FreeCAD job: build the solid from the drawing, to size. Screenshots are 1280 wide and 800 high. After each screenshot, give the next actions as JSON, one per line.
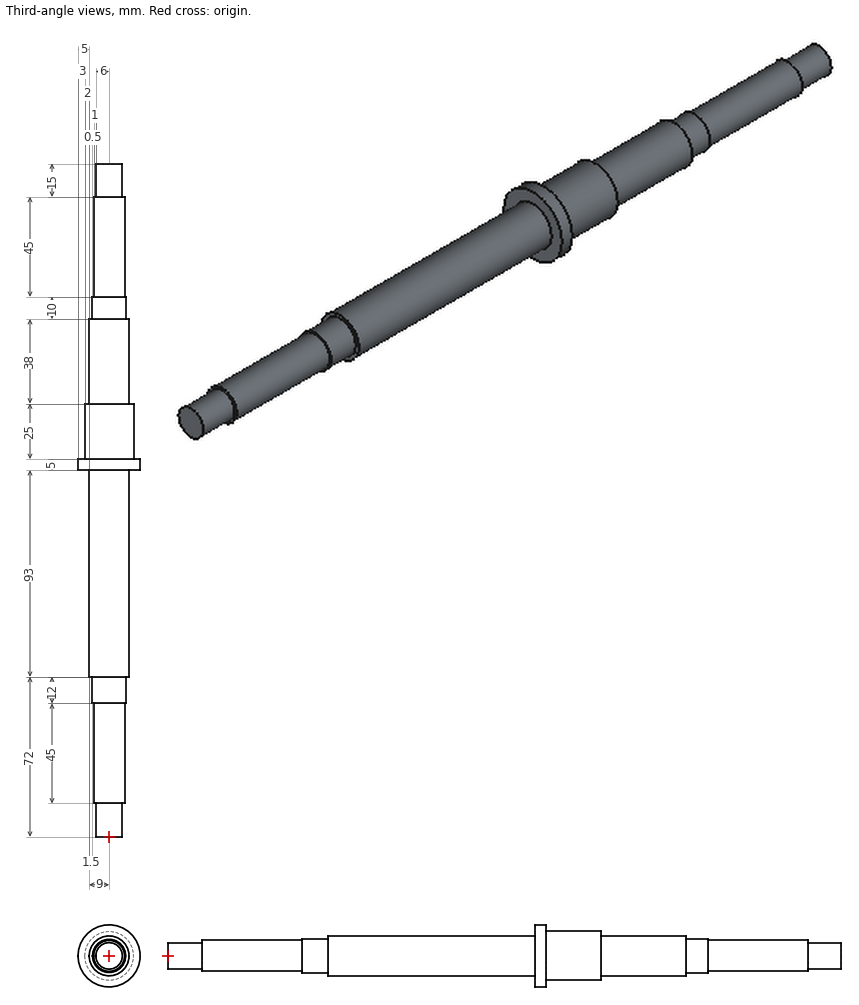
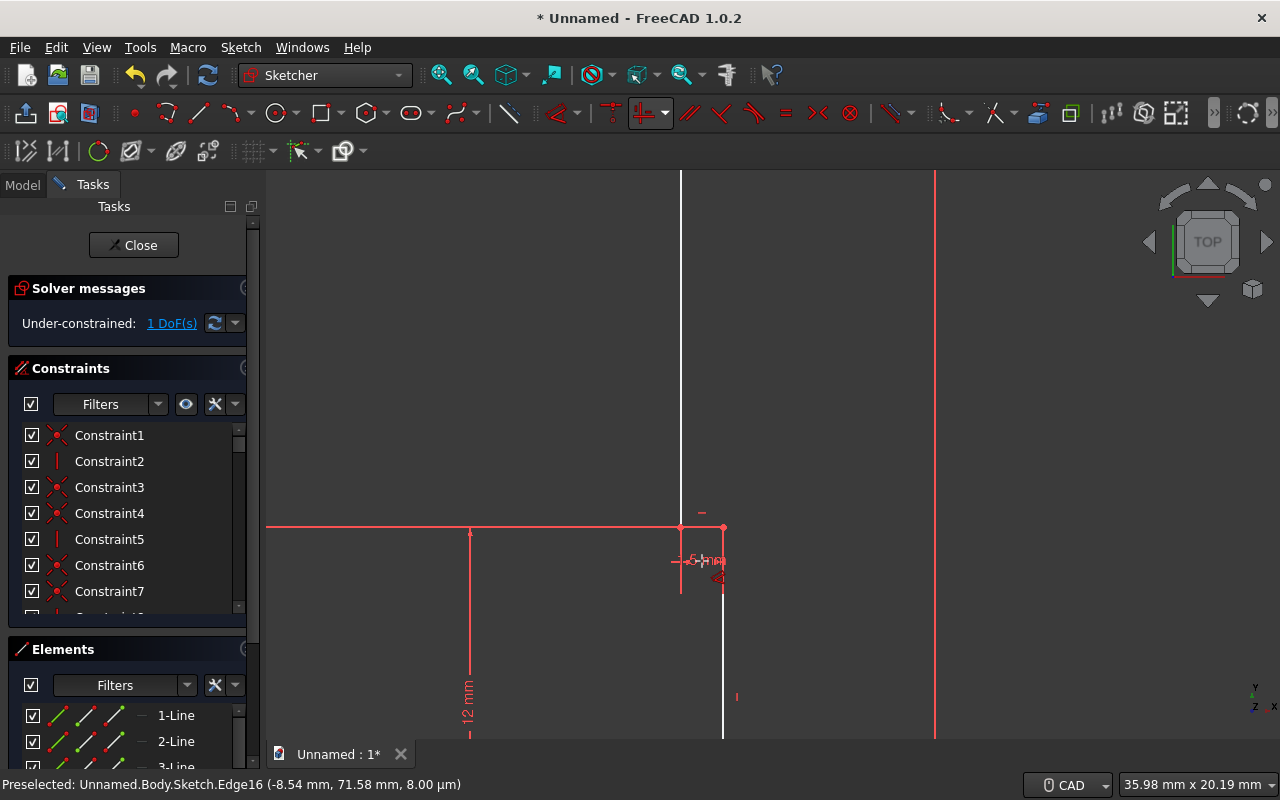
{"action": "scroll", "coordinate": [703, 569], "scroll_direction": "down", "scroll_amount": 15}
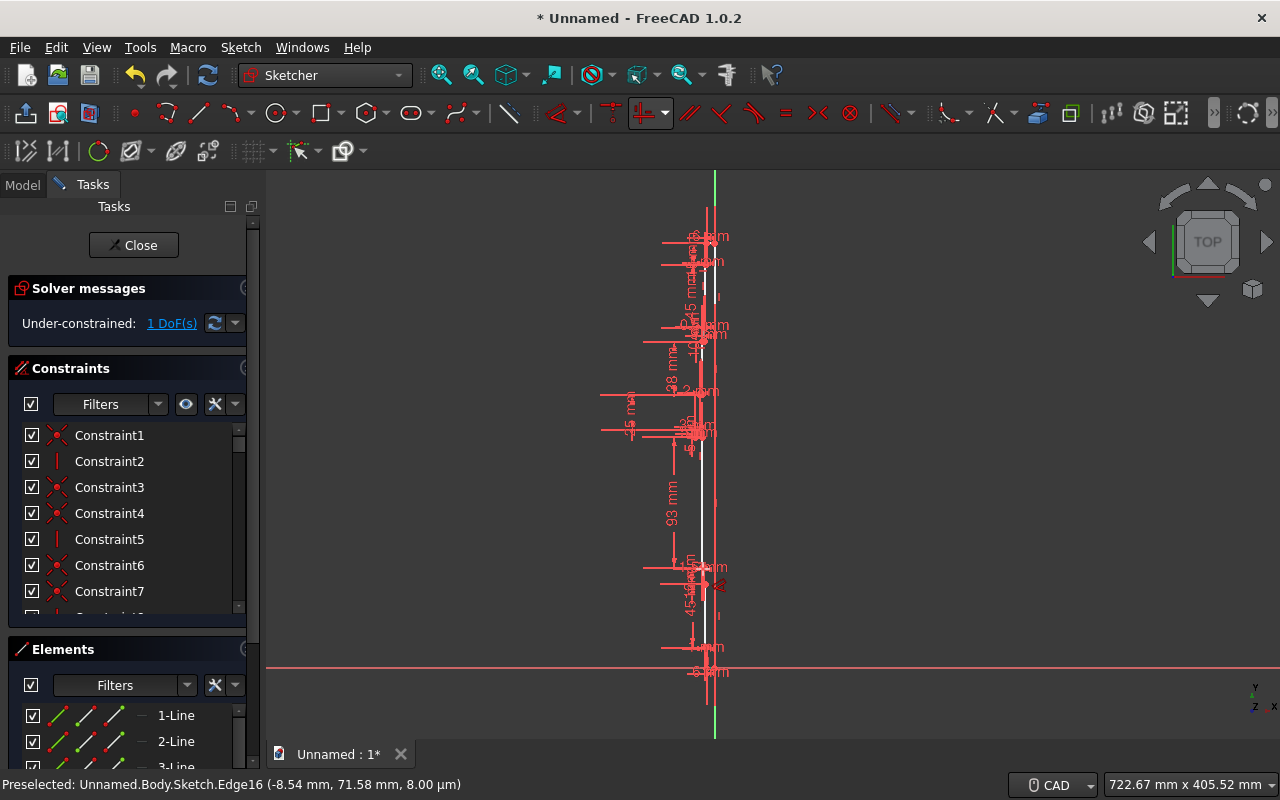
{"action": "scroll", "coordinate": [702, 568], "scroll_direction": "up", "scroll_amount": 9}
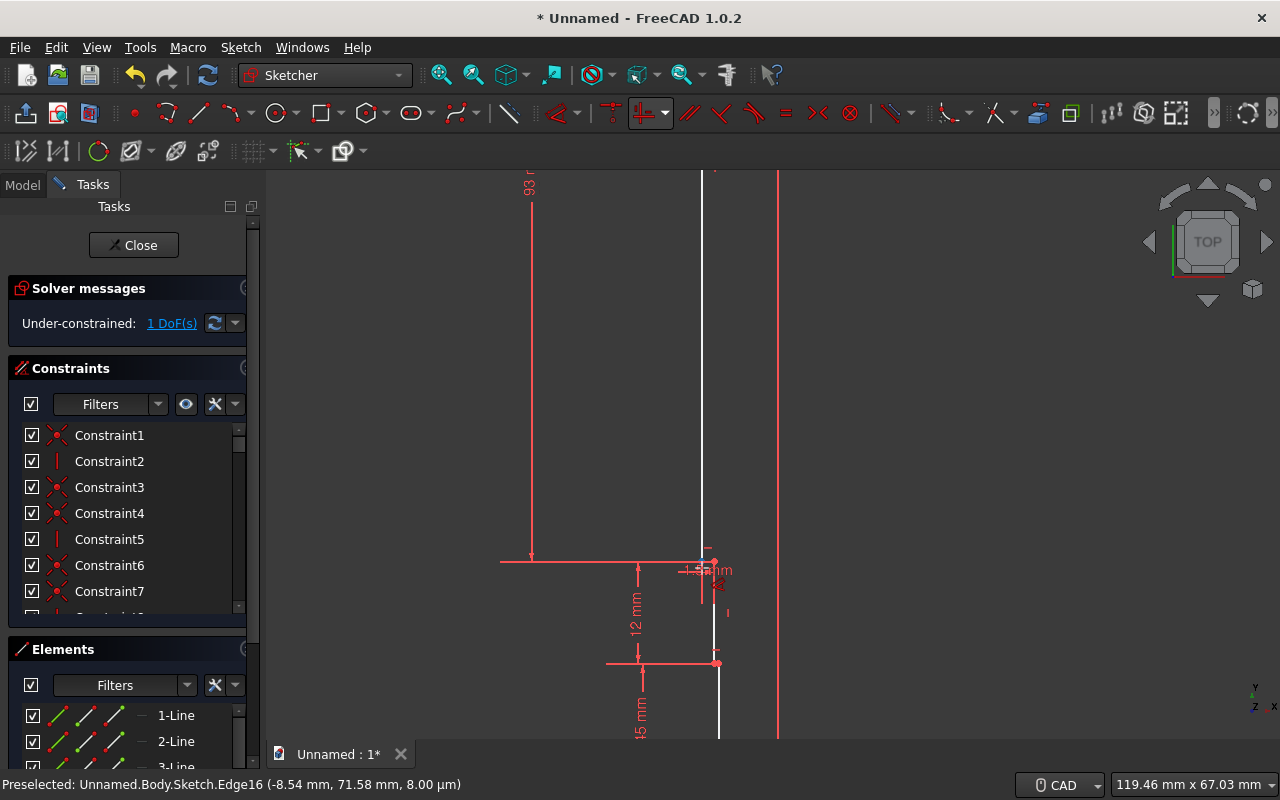
{"action": "left_click", "coordinate": [702, 562]}
{"action": "left_click", "coordinate": [812, 636]}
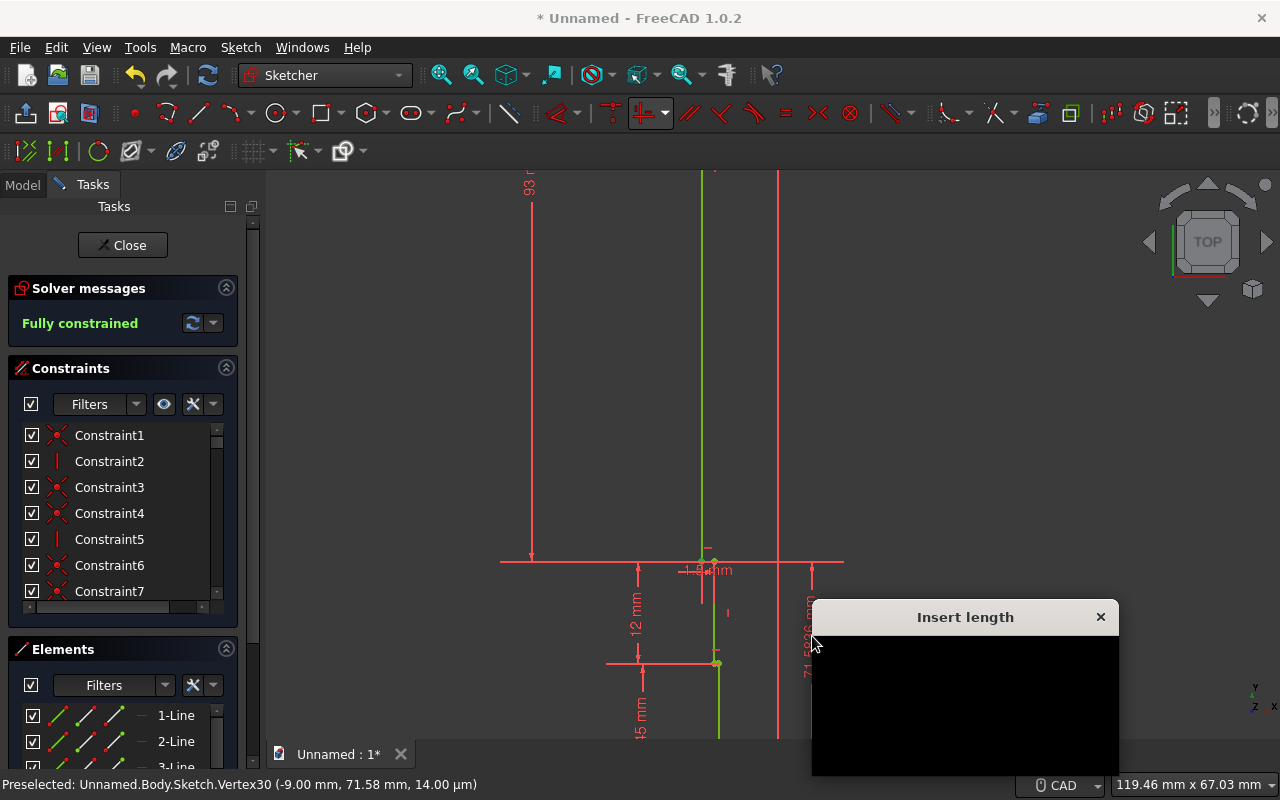
{"action": "type", "text": "72"}
{"action": "key", "text": "Return"}
{"action": "key", "text": "Escape"}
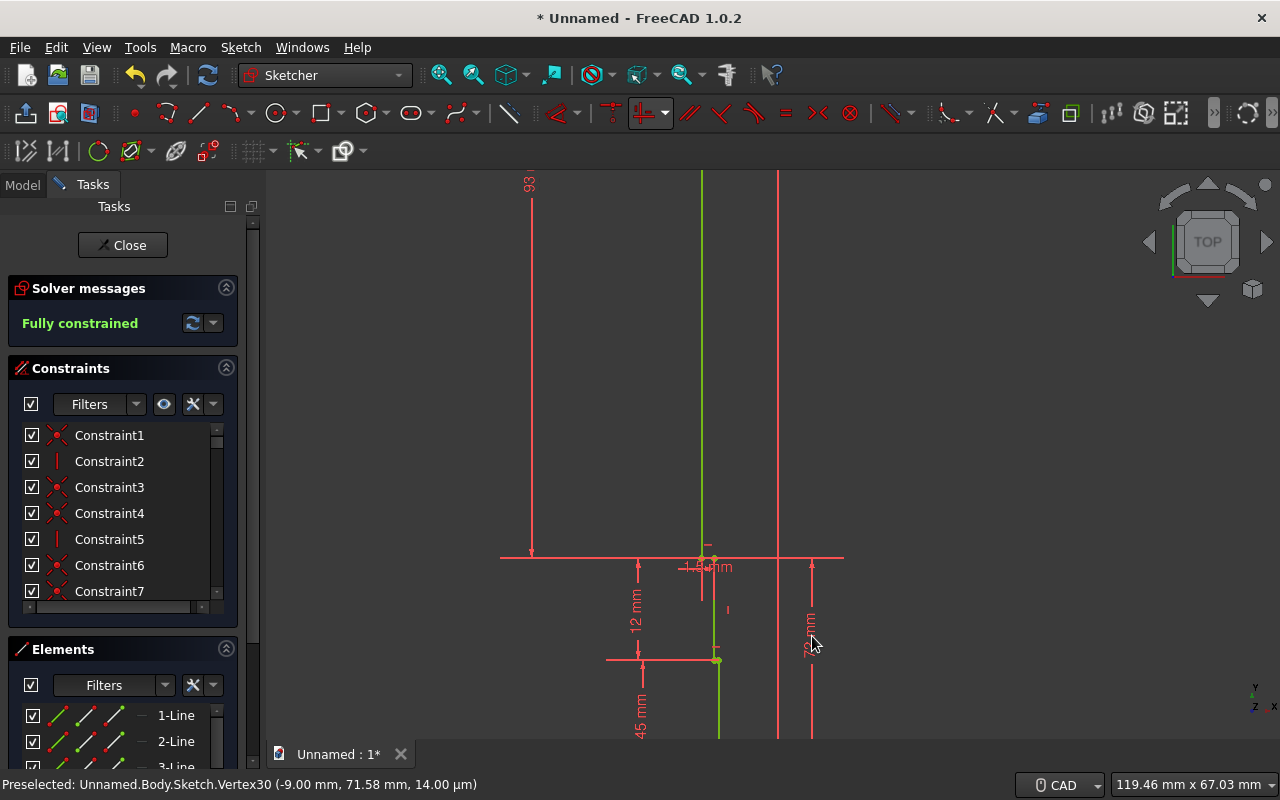
{"action": "left_click", "coordinate": [123, 245]}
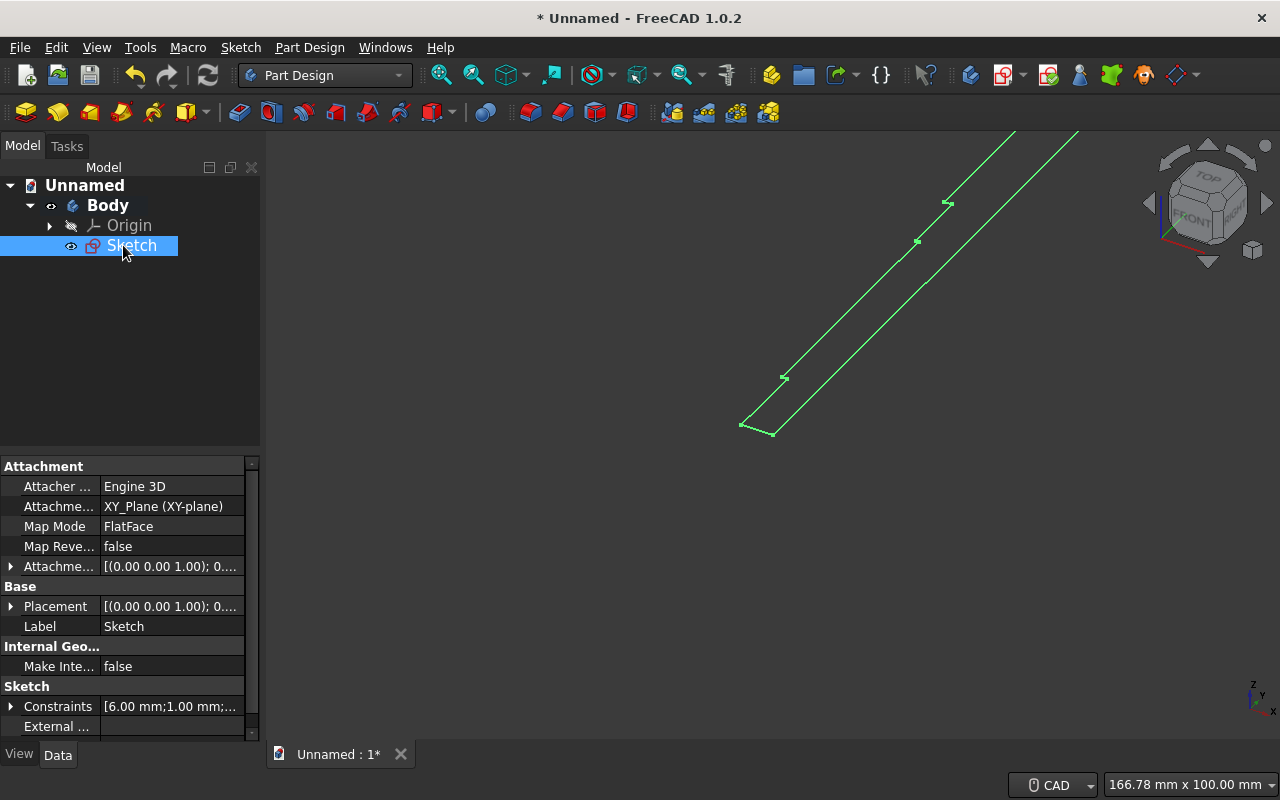
{"action": "left_click", "coordinate": [58, 112]}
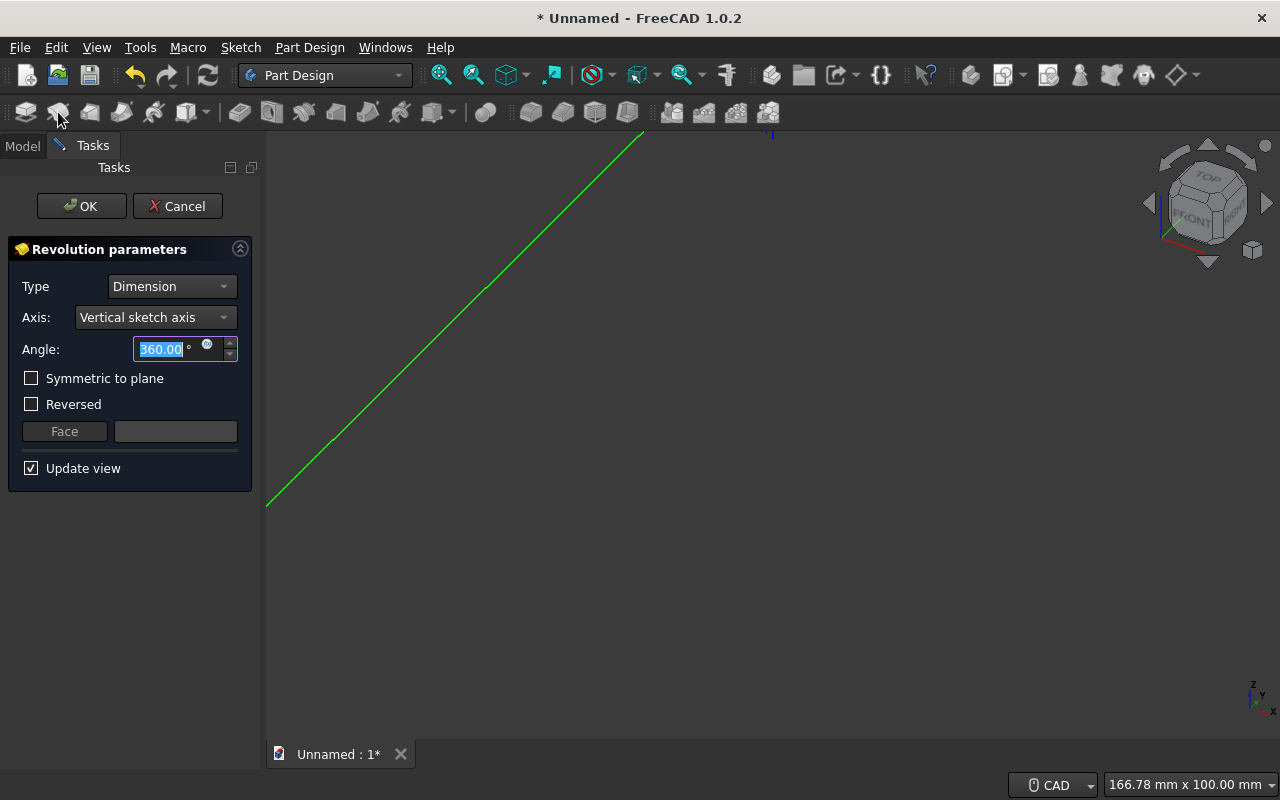
{"action": "left_click", "coordinate": [82, 206]}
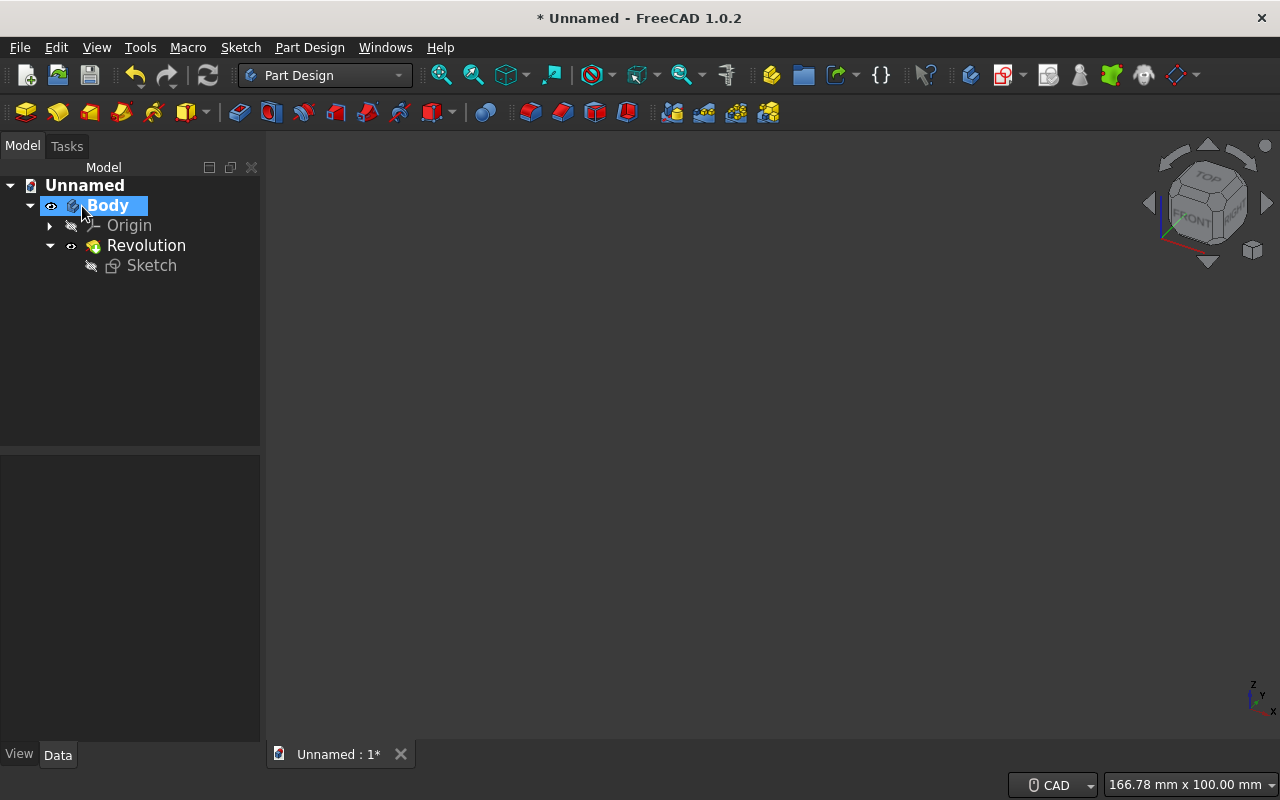
{"action": "key", "text": "0"}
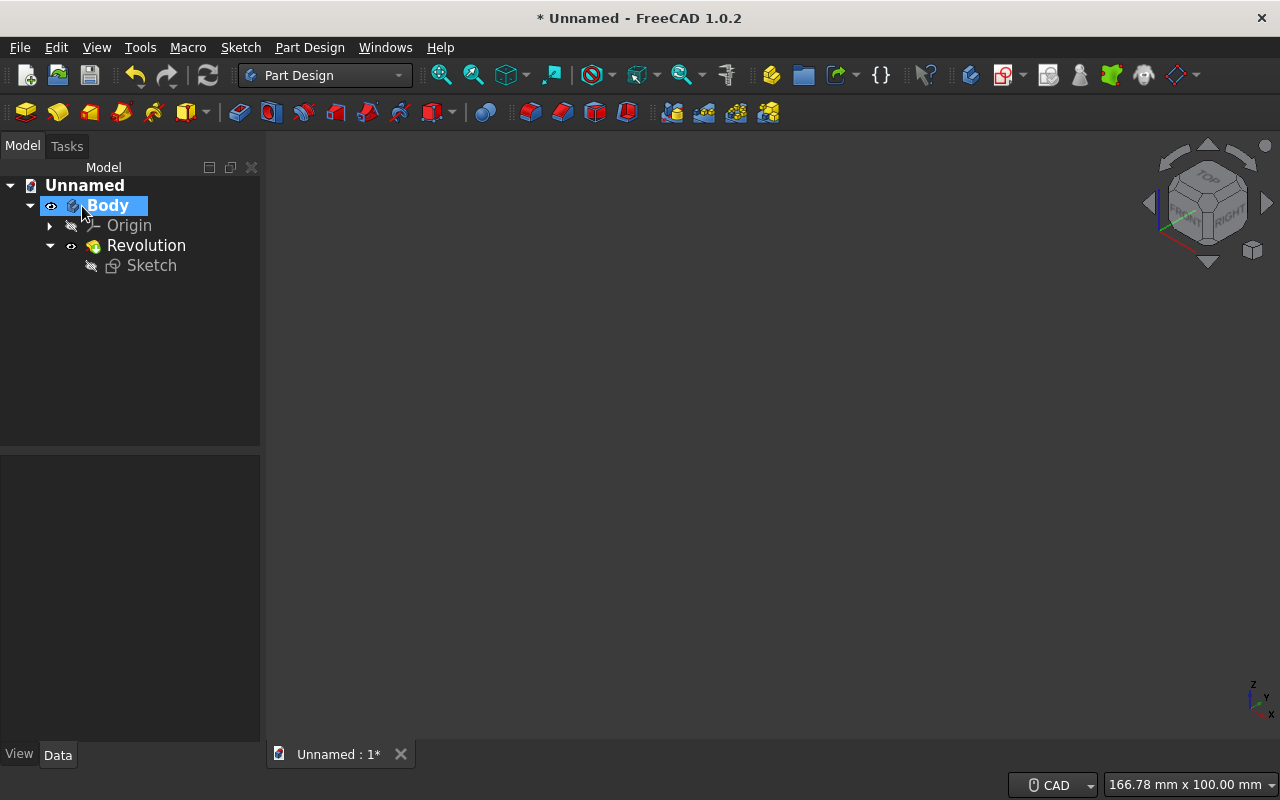
{"action": "key", "text": "v f"}